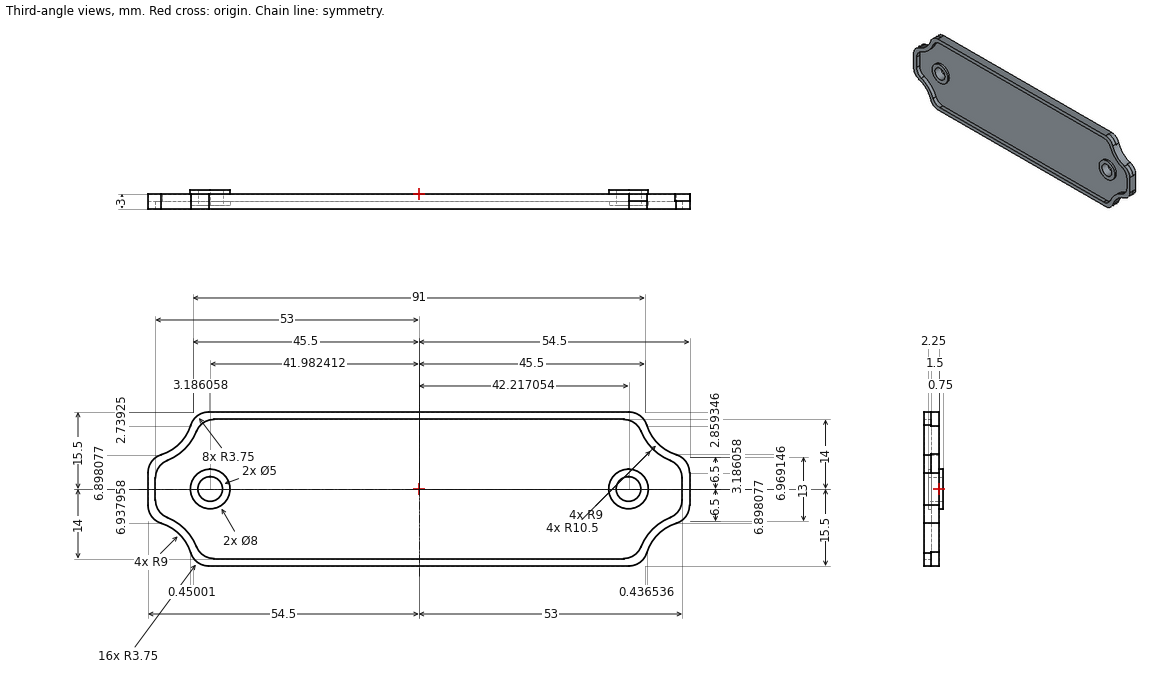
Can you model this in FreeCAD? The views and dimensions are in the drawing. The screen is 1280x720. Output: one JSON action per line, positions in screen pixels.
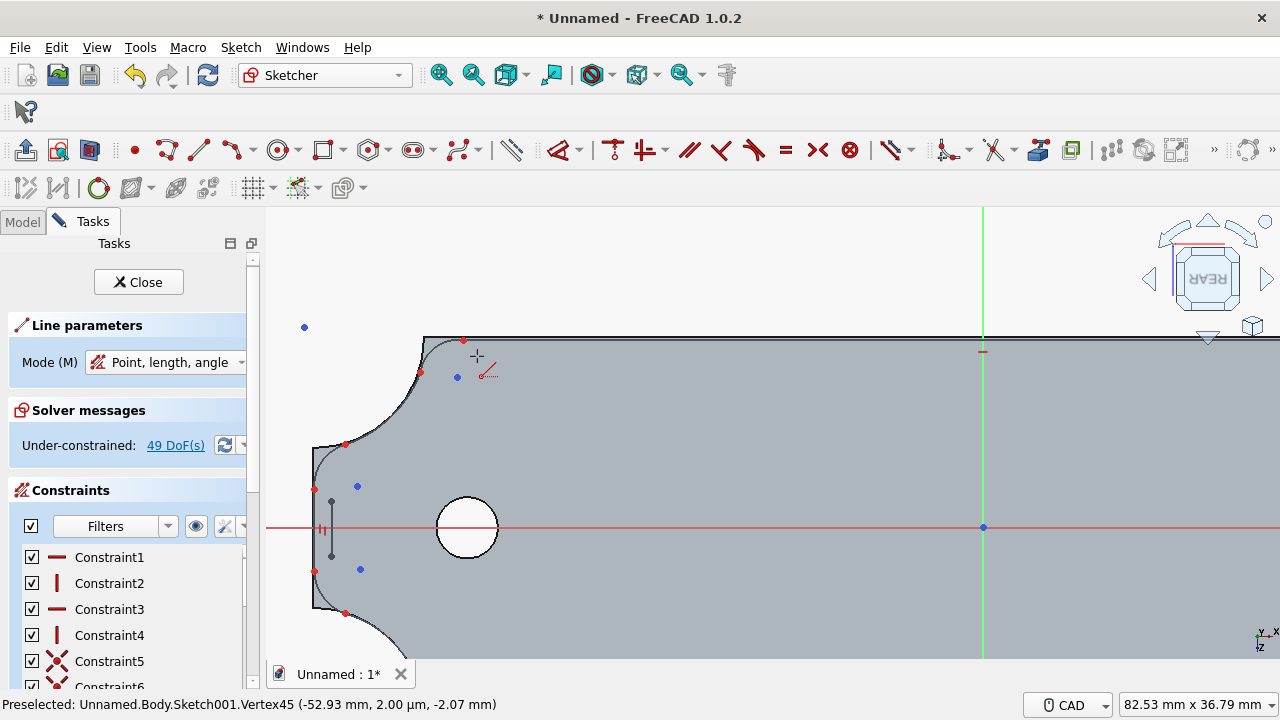
{"action": "left_click", "coordinate": [476, 356]}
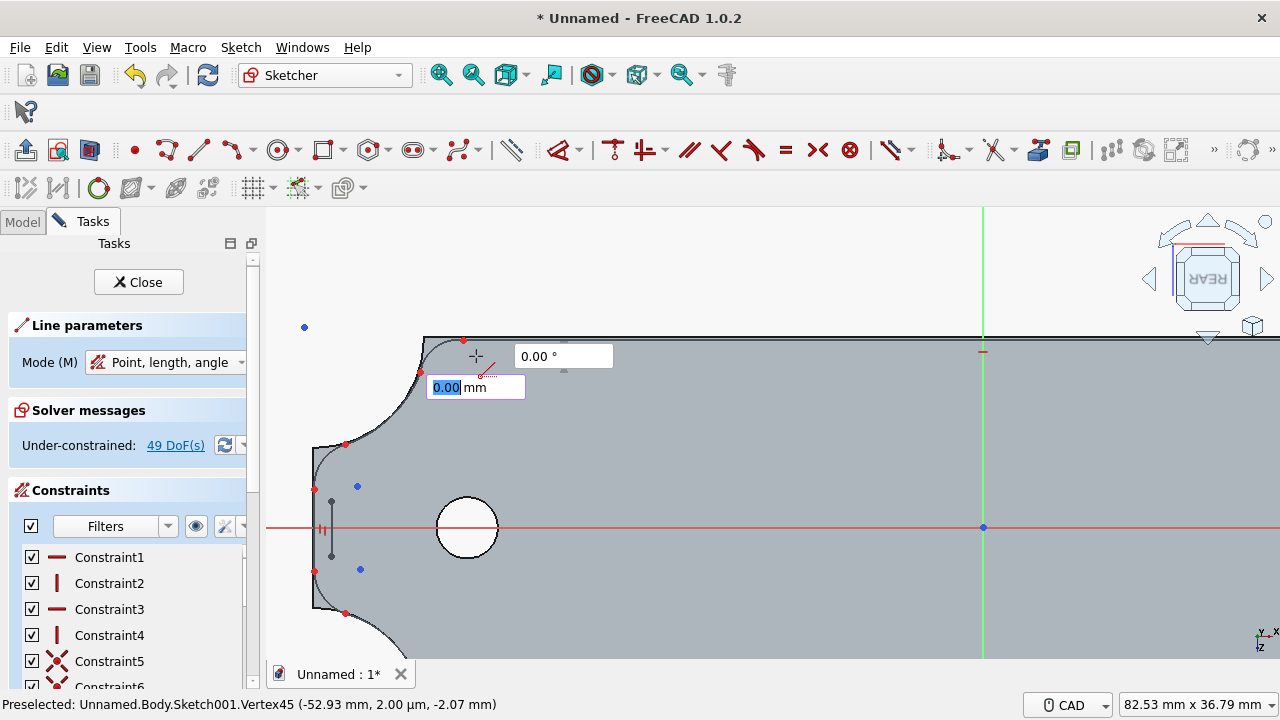
{"action": "scroll", "coordinate": [477, 356], "scroll_direction": "down", "scroll_amount": 4}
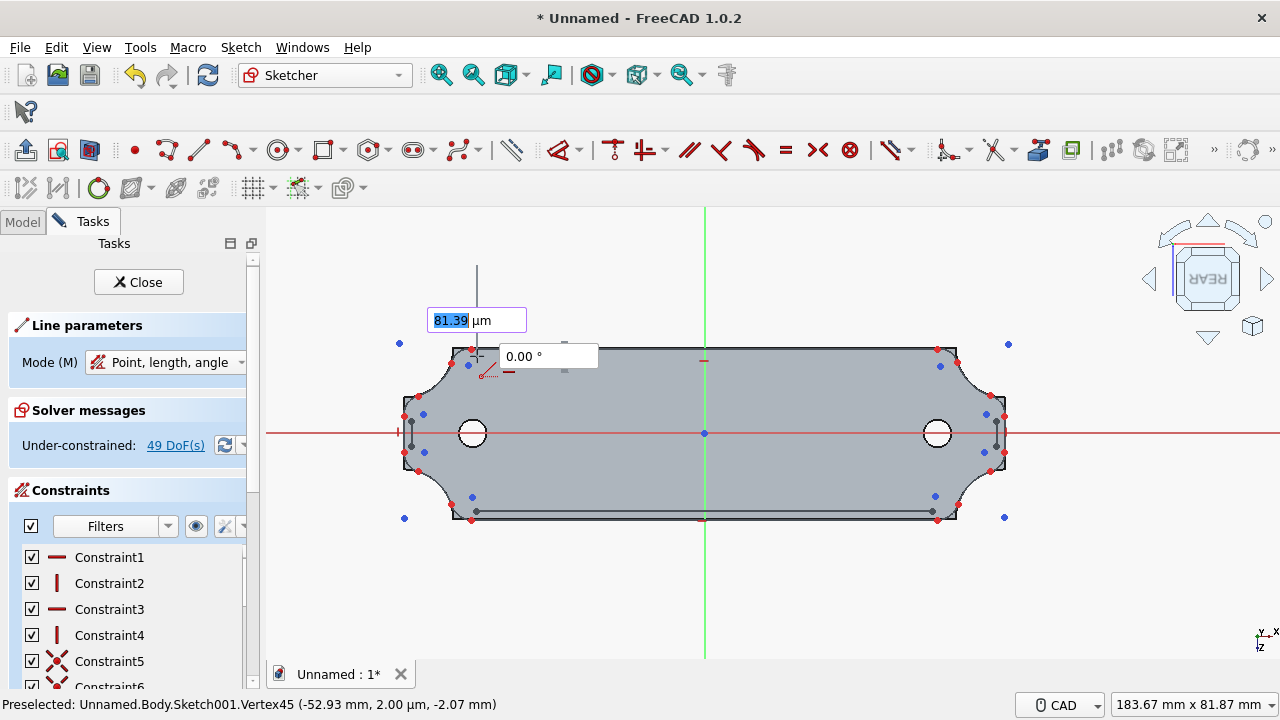
{"action": "scroll", "coordinate": [932, 356], "scroll_direction": "up", "scroll_amount": 4}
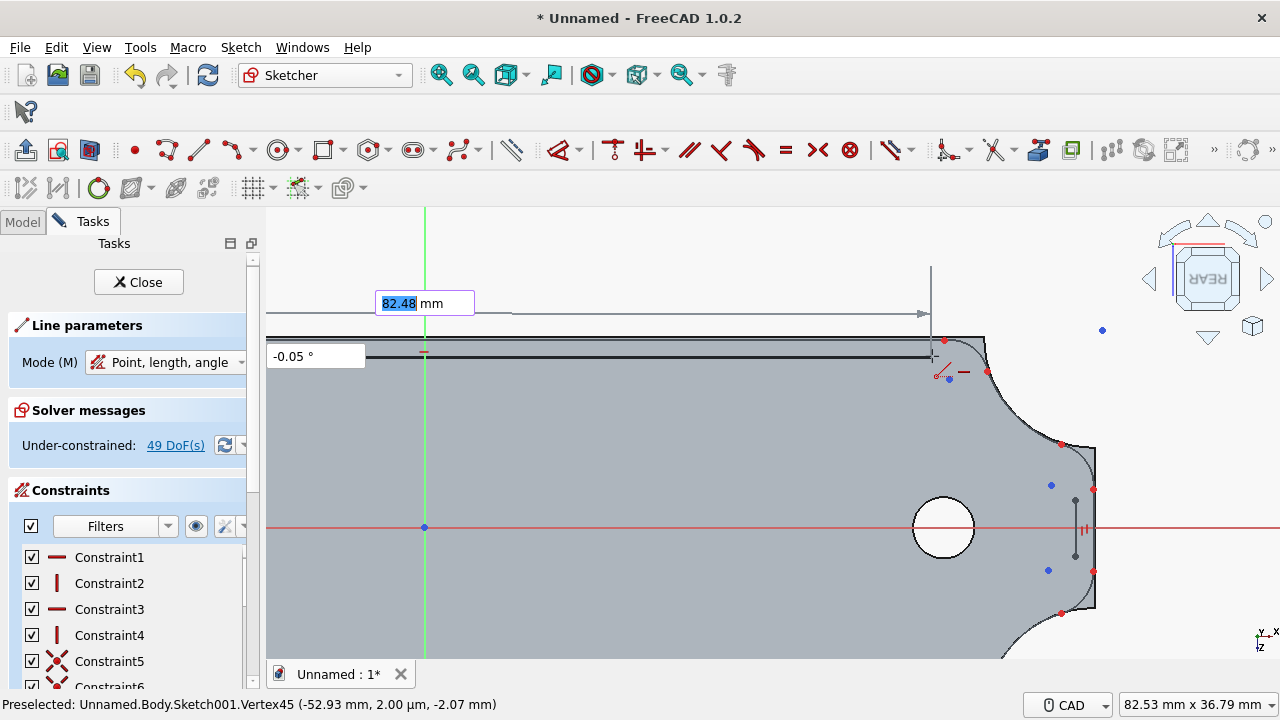
{"action": "left_click", "coordinate": [932, 356]}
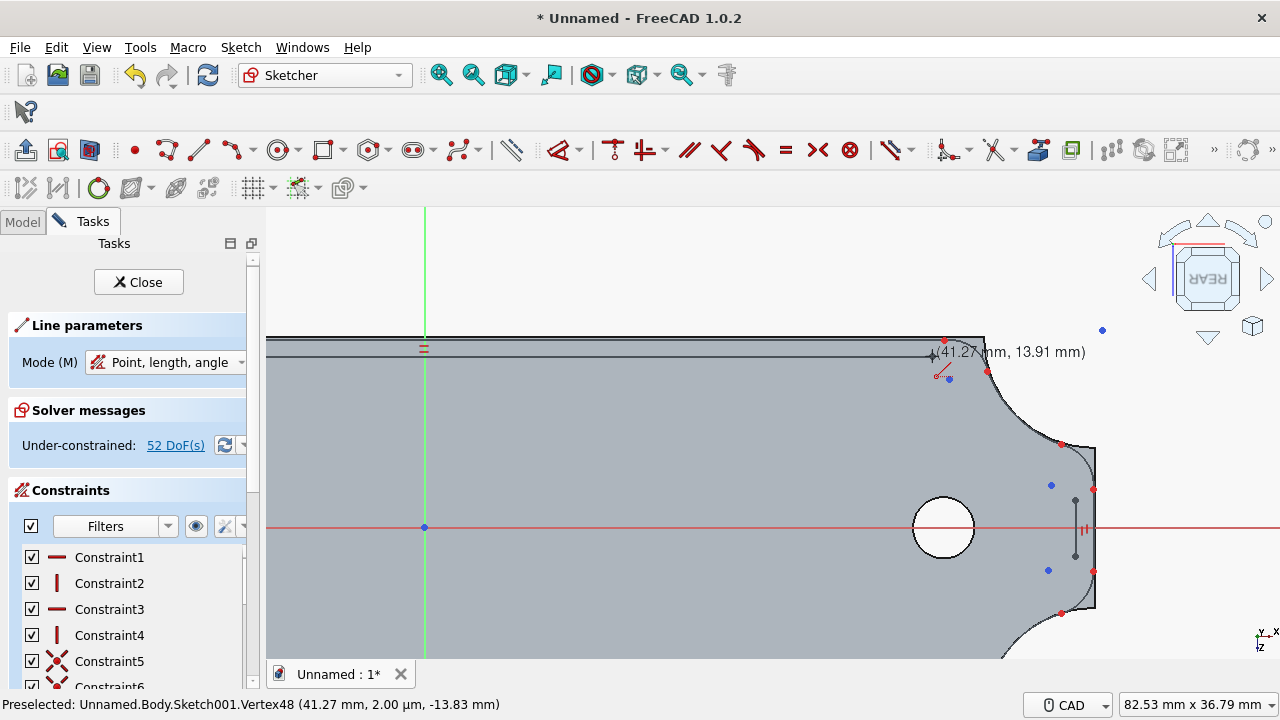
{"action": "left_click", "coordinate": [232, 150]}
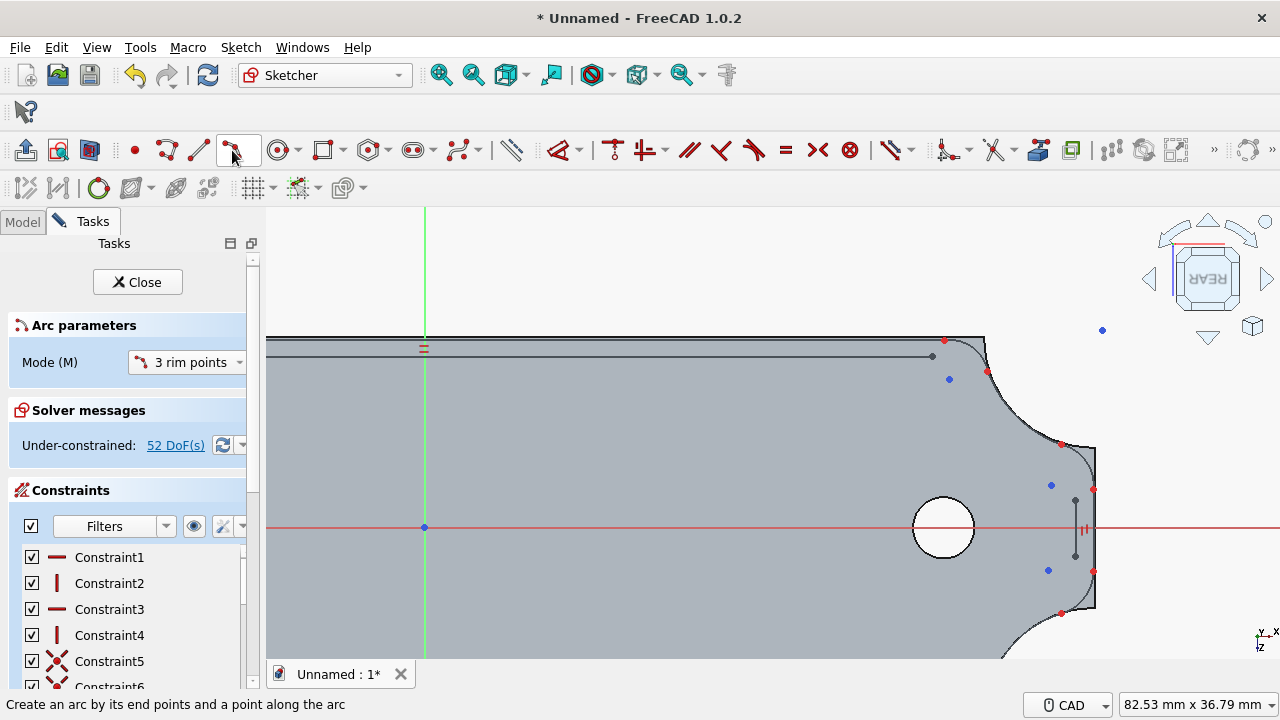
{"action": "left_click", "coordinate": [1076, 557]}
{"action": "left_click", "coordinate": [1047, 598]}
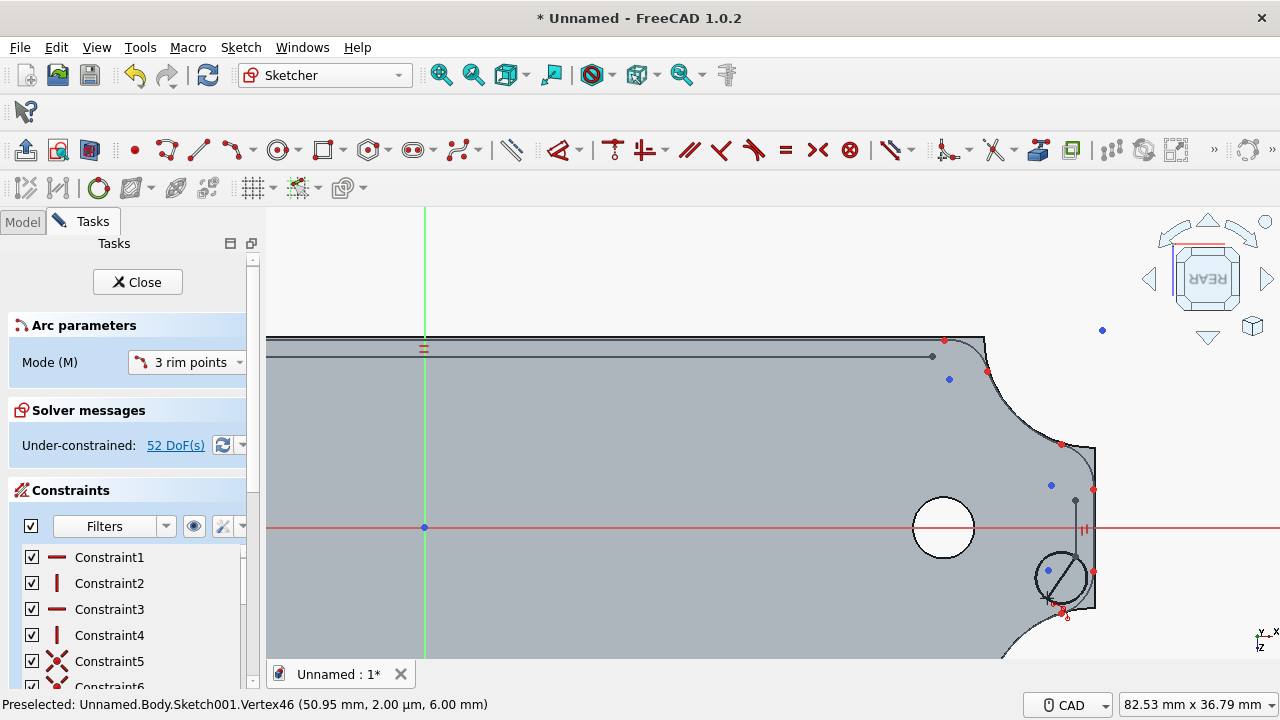
{"action": "scroll", "coordinate": [1068, 581], "scroll_direction": "up", "scroll_amount": 4}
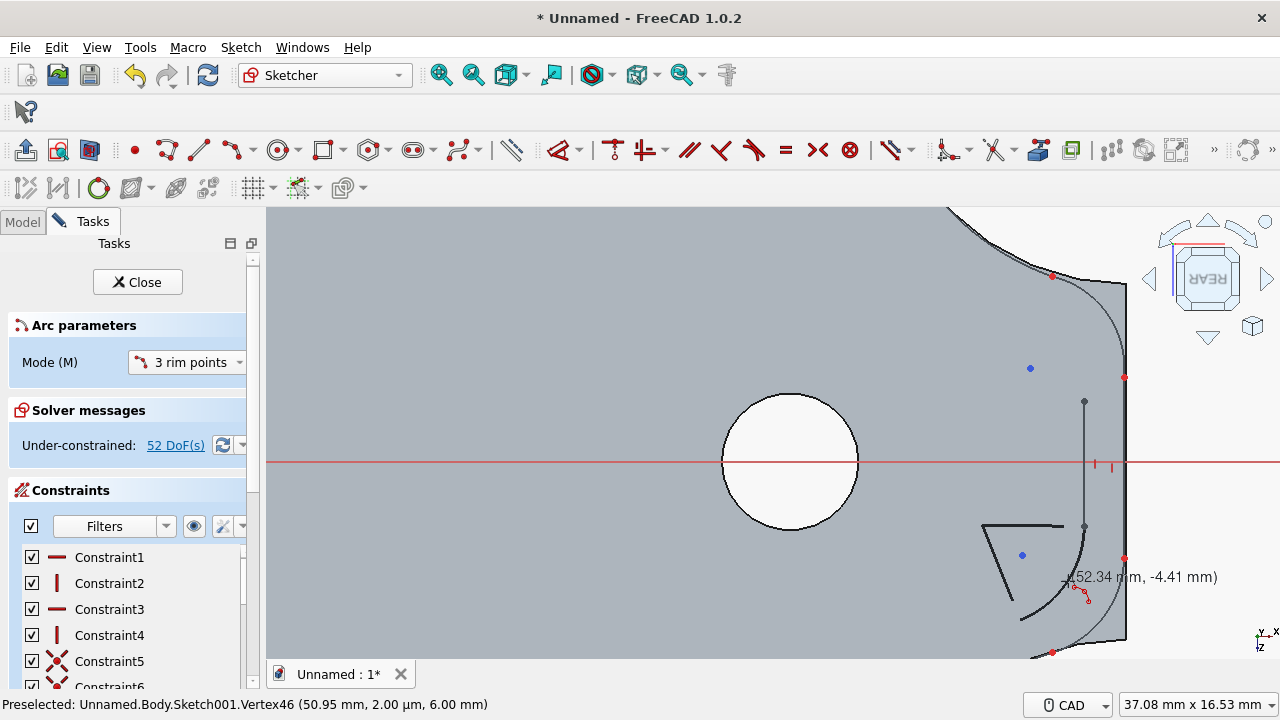
{"action": "left_click", "coordinate": [1067, 581]}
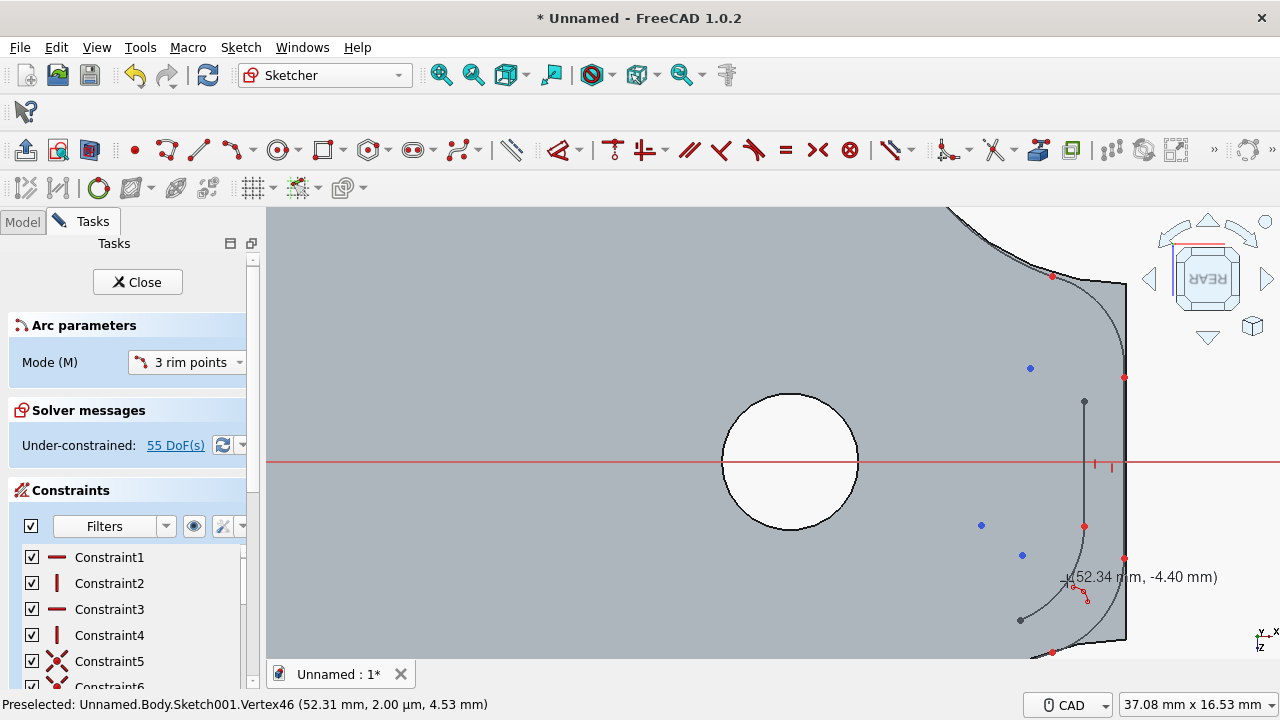
{"action": "left_click", "coordinate": [1020, 620]}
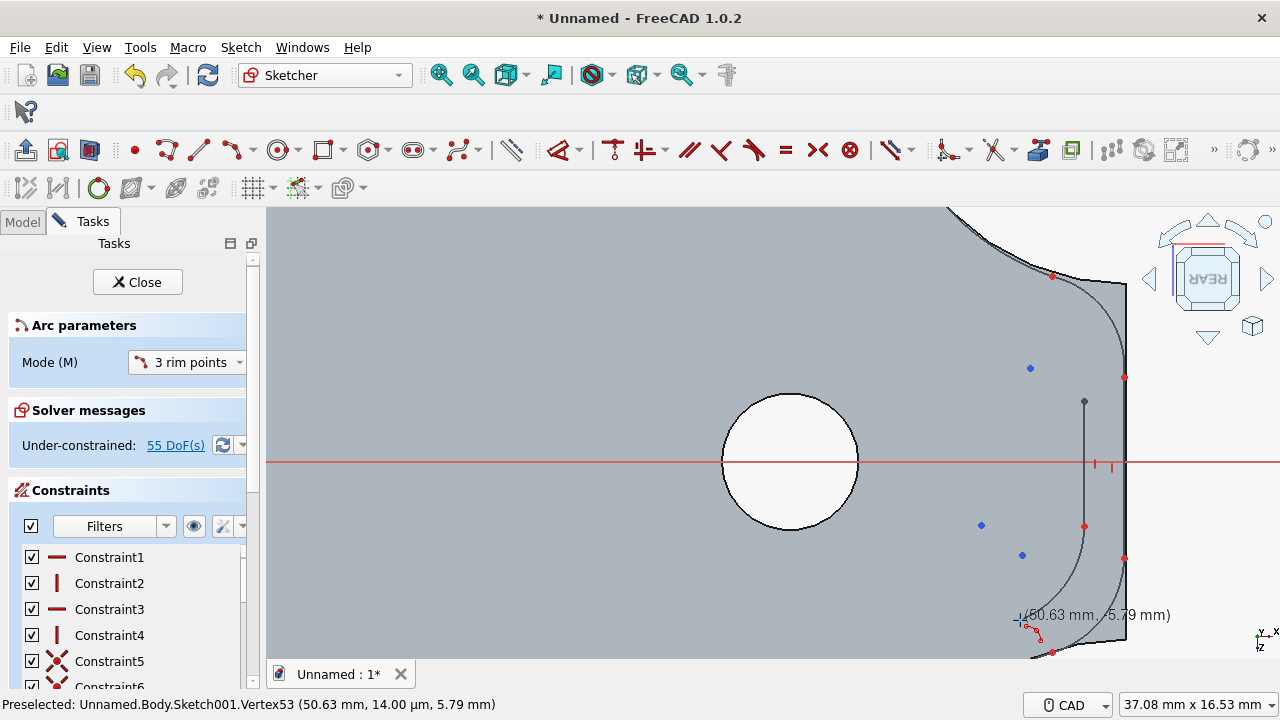
{"action": "scroll", "coordinate": [975, 426], "scroll_direction": "down", "scroll_amount": 8}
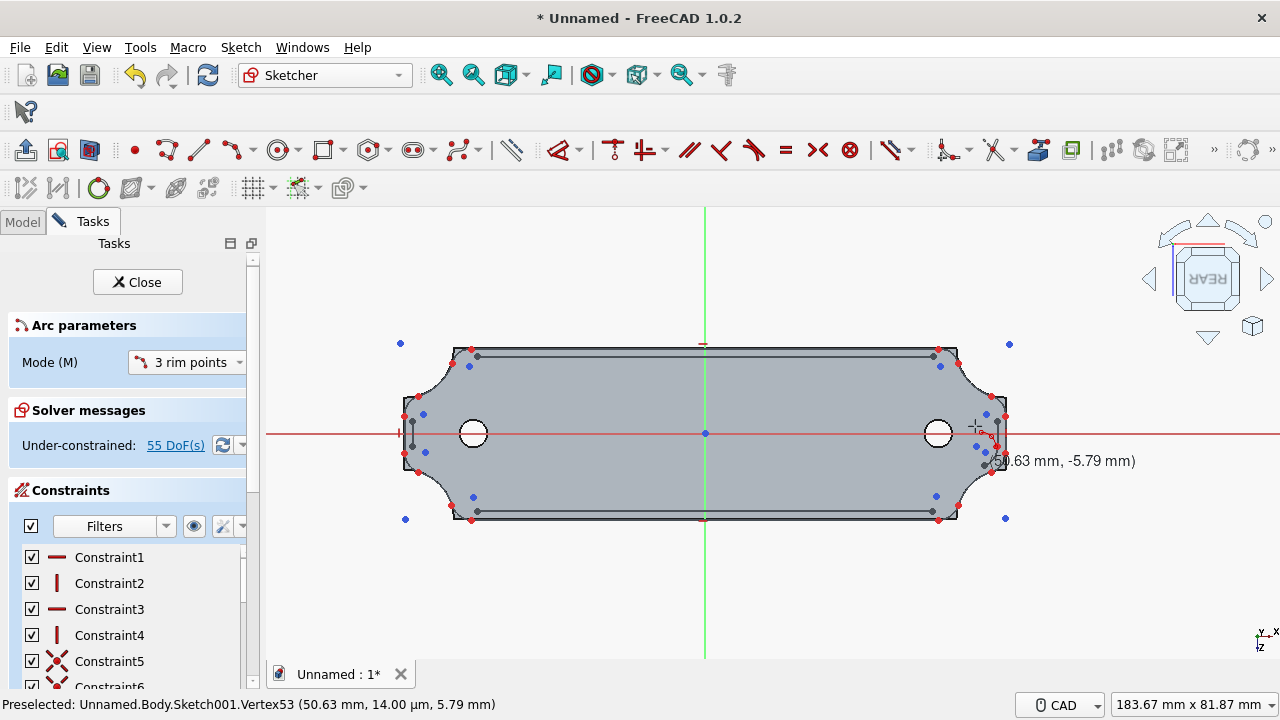
{"action": "scroll", "coordinate": [952, 498], "scroll_direction": "up", "scroll_amount": 4}